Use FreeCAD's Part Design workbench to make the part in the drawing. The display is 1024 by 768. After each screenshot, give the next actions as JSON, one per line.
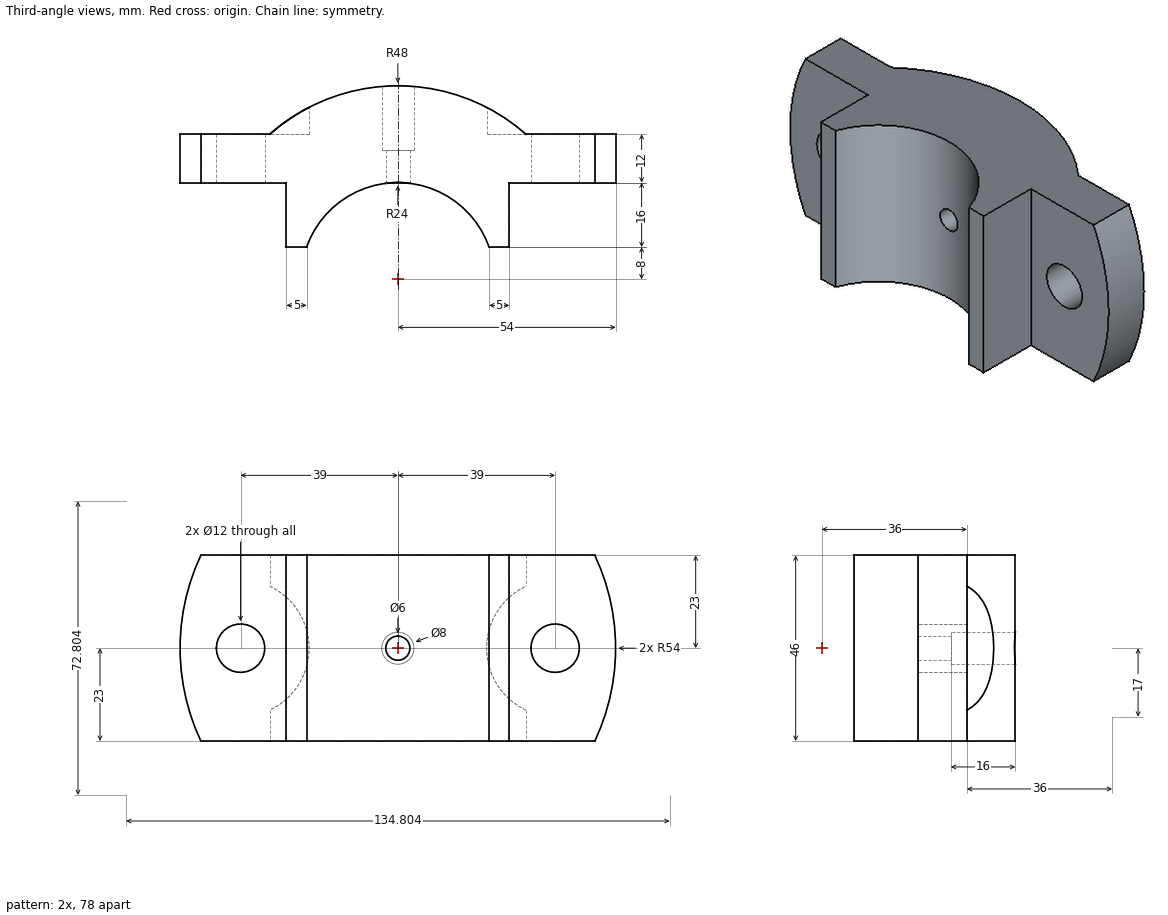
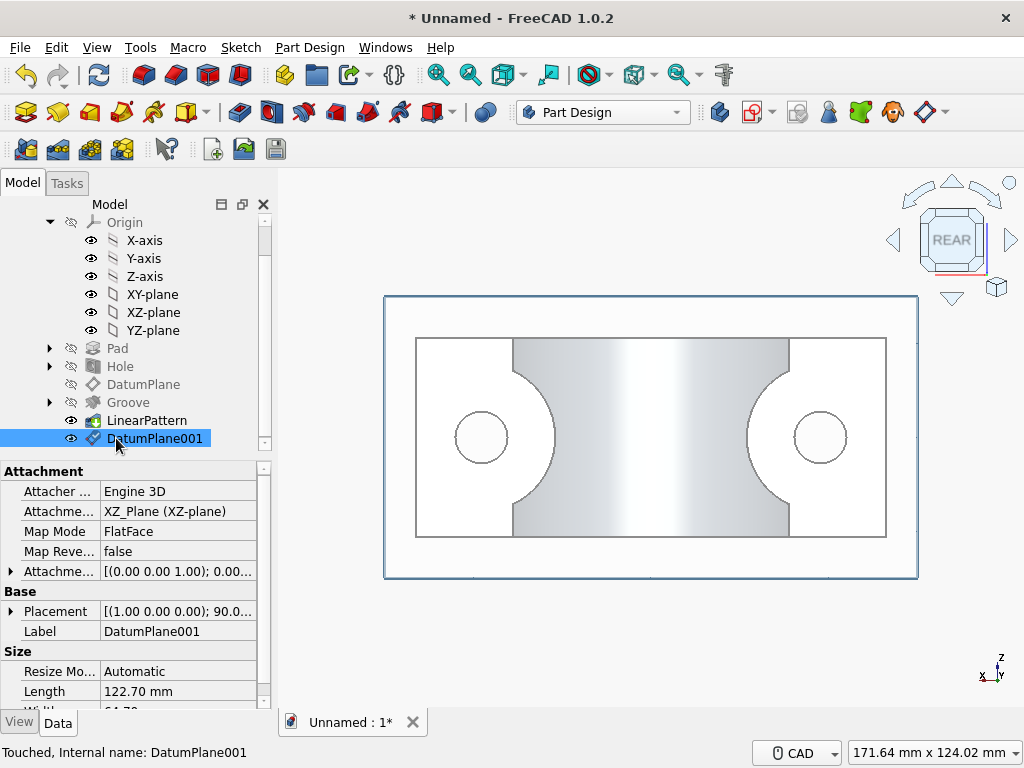
{"action": "left_click", "coordinate": [752, 112]}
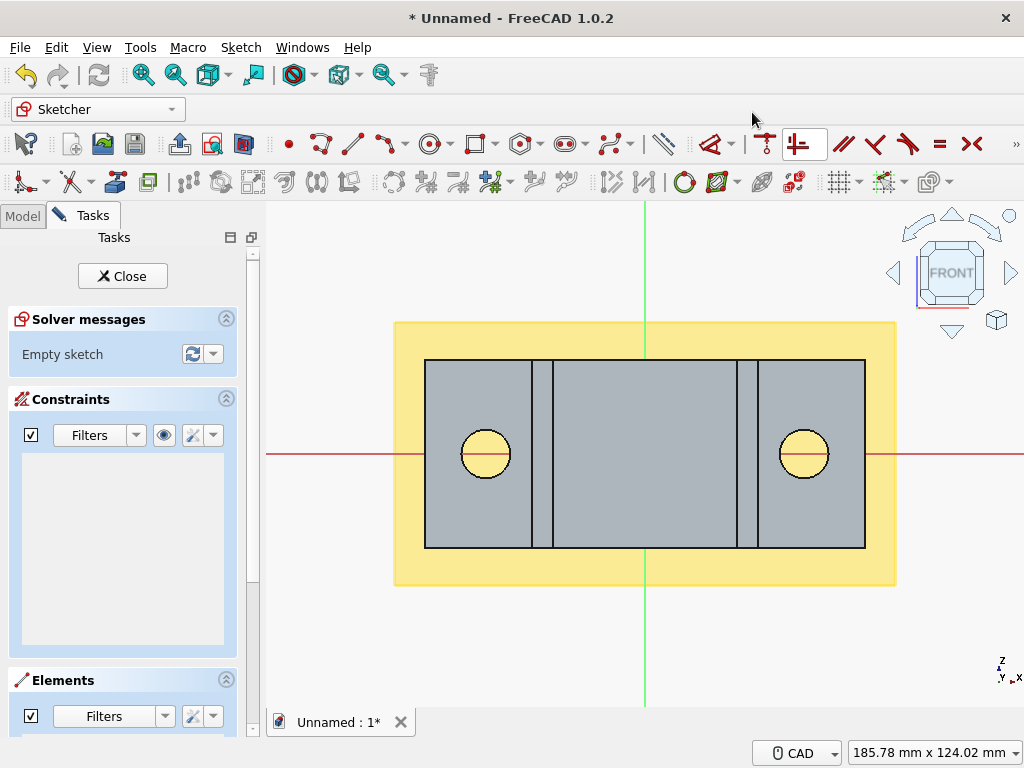
{"action": "left_click", "coordinate": [244, 144]}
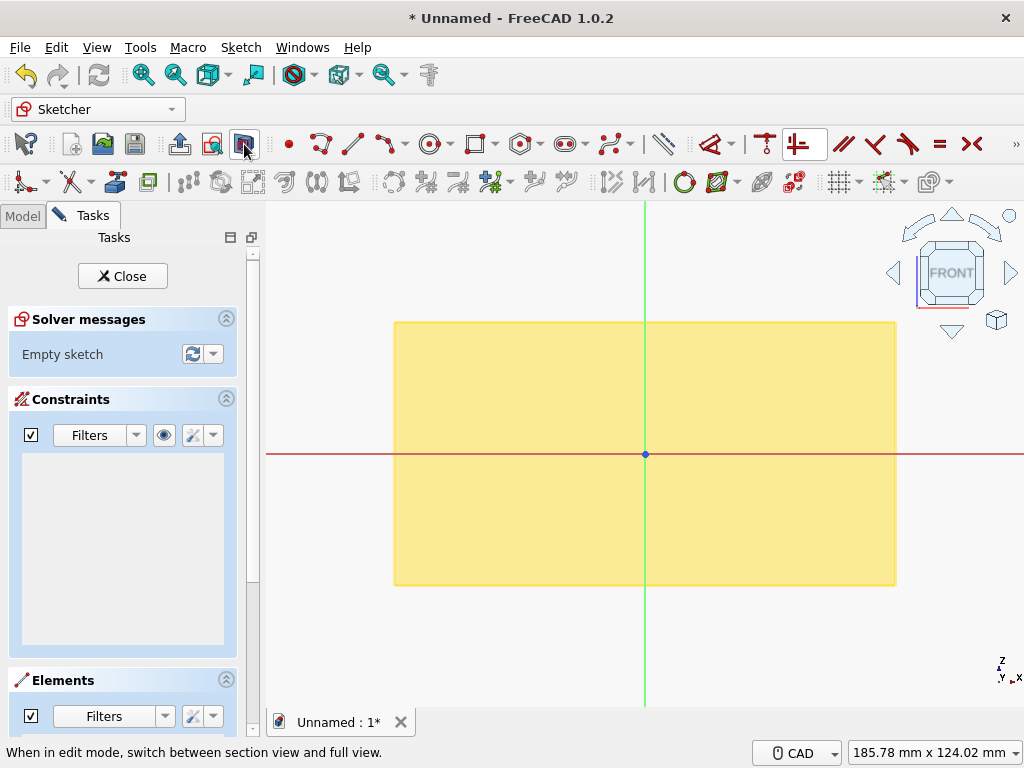
{"action": "scroll", "coordinate": [654, 454], "scroll_direction": "up", "scroll_amount": 11}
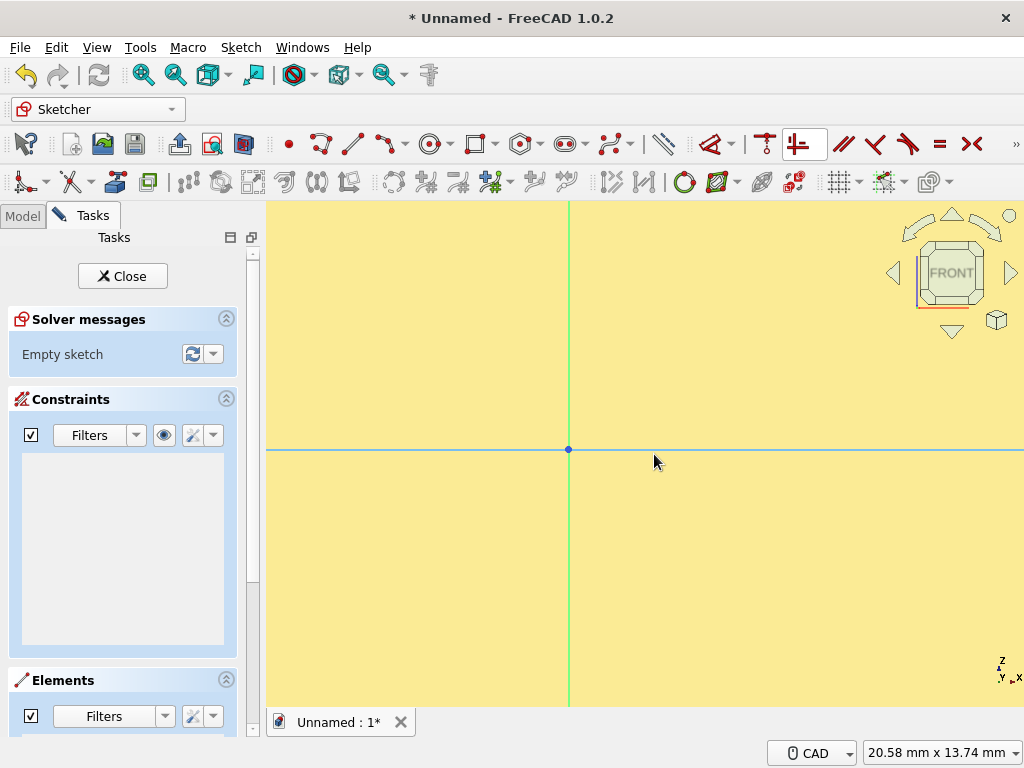
{"action": "left_click", "coordinate": [430, 144]}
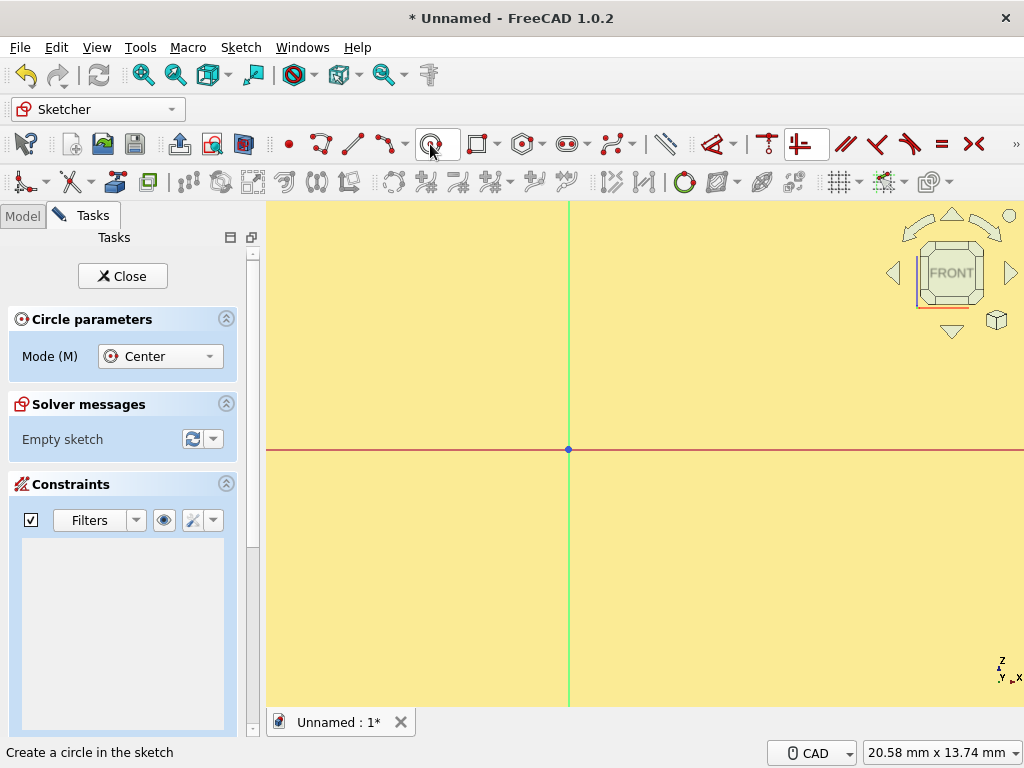
{"action": "left_click", "coordinate": [569, 450]}
{"action": "mouse_move", "coordinate": [673, 346]}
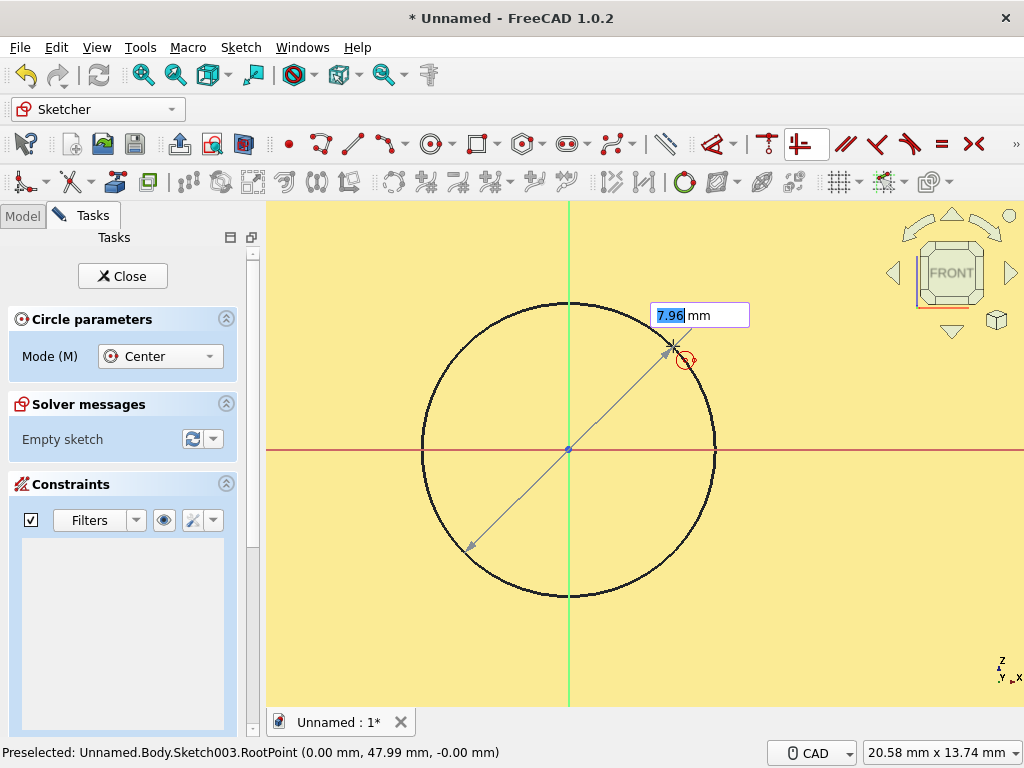
{"action": "type", "text": "8"}
{"action": "key", "text": "Return"}
{"action": "key", "text": "Escape"}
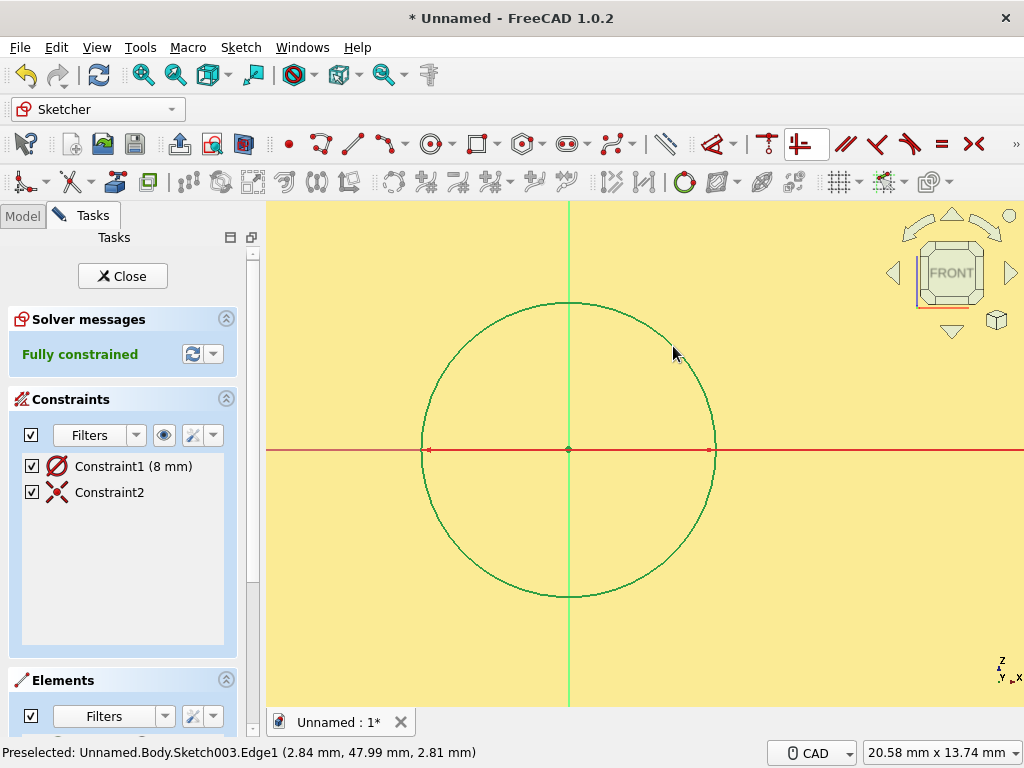
{"action": "left_click", "coordinate": [123, 276]}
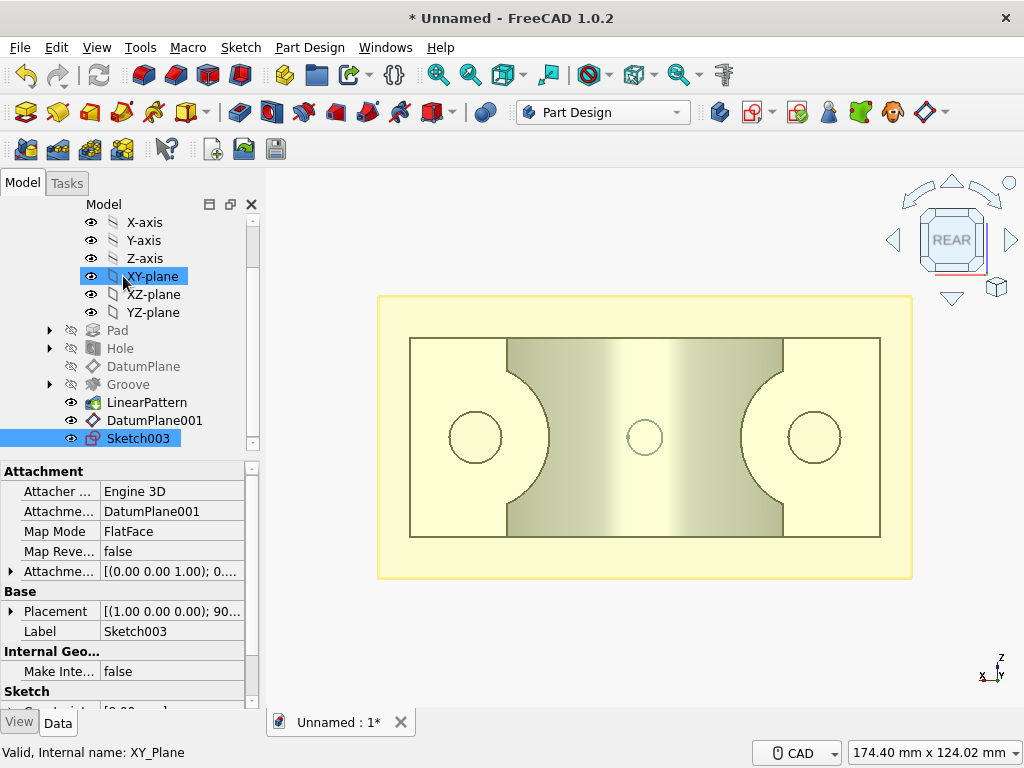
{"action": "left_click", "coordinate": [240, 112]}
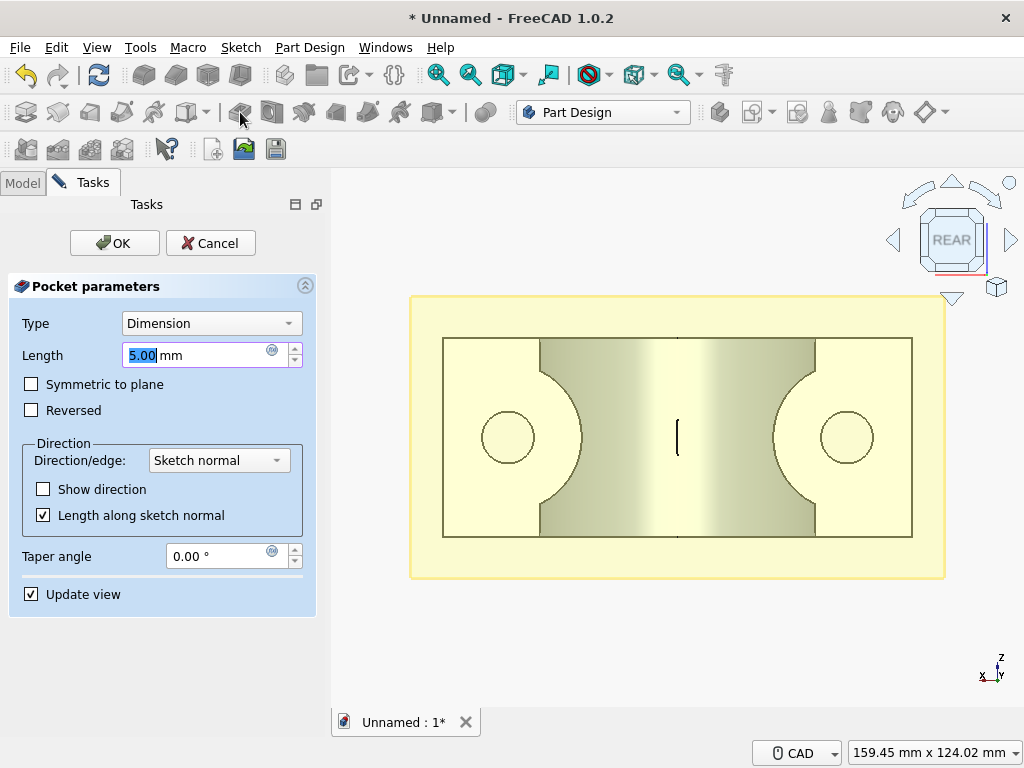
{"action": "type", "text": "16"}
{"action": "key", "text": "Tab"}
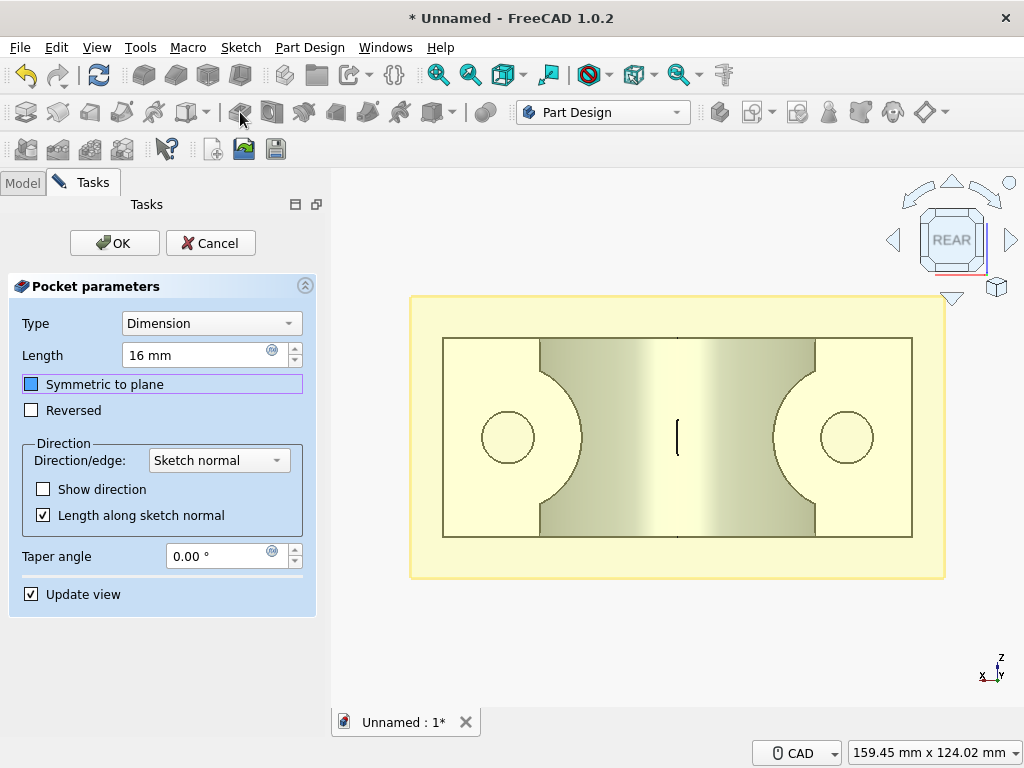
{"action": "left_click", "coordinate": [30, 410]}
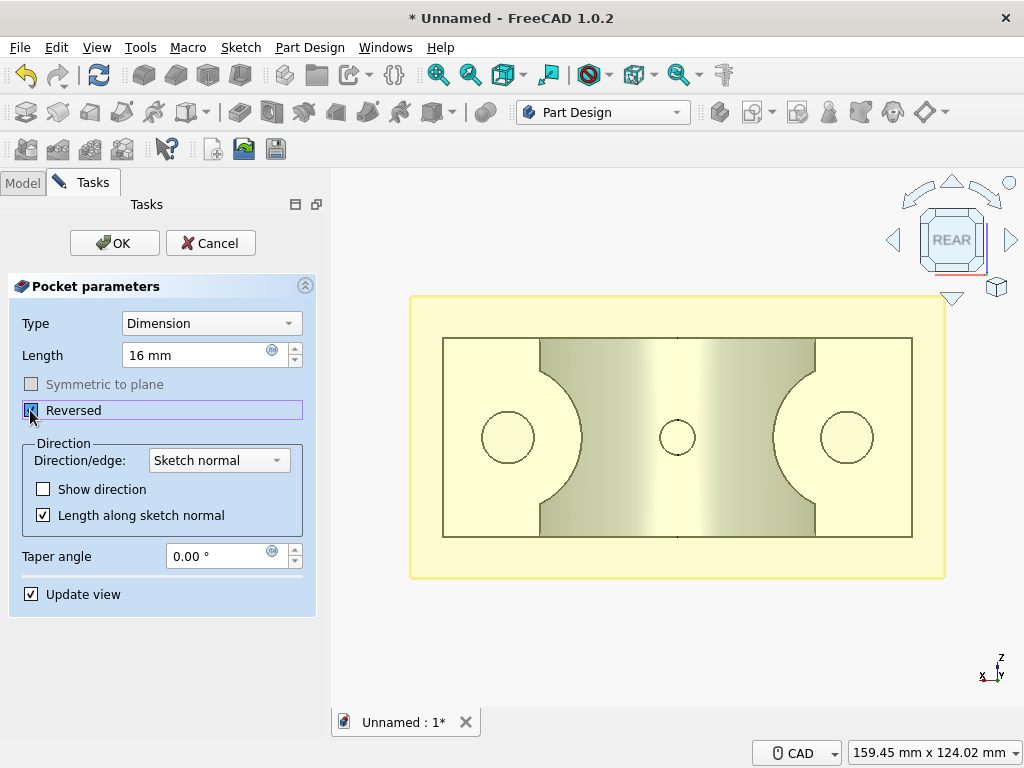
{"action": "left_click", "coordinate": [115, 243]}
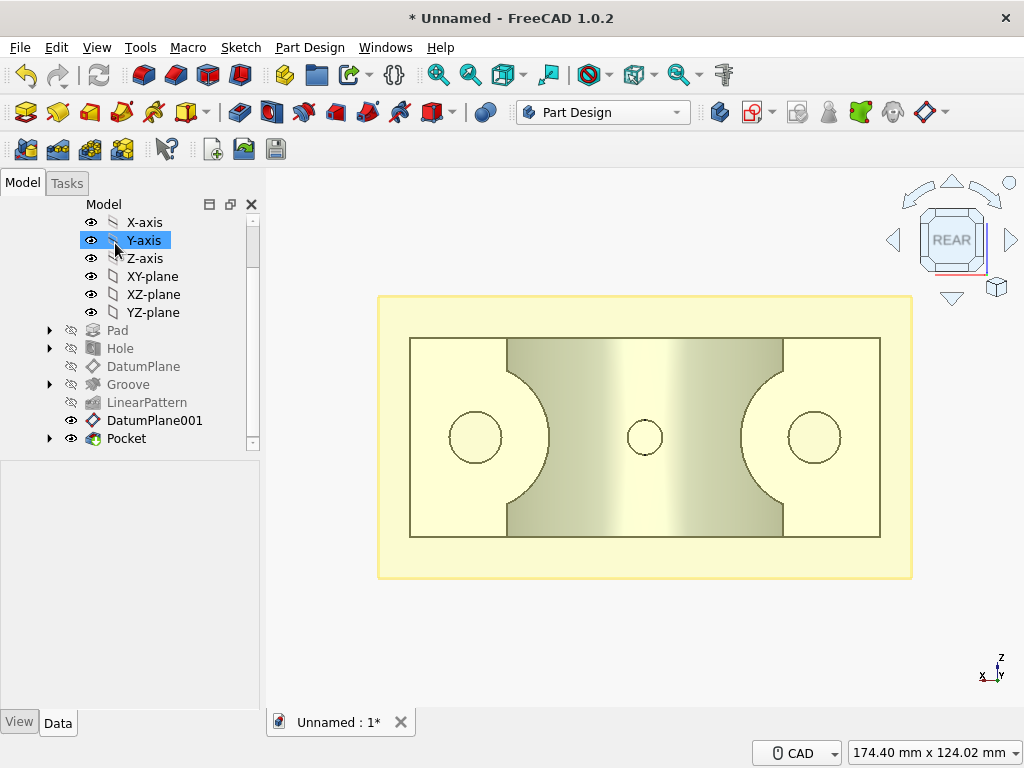
{"action": "left_click", "coordinate": [116, 420]}
{"action": "key", "text": "space"}